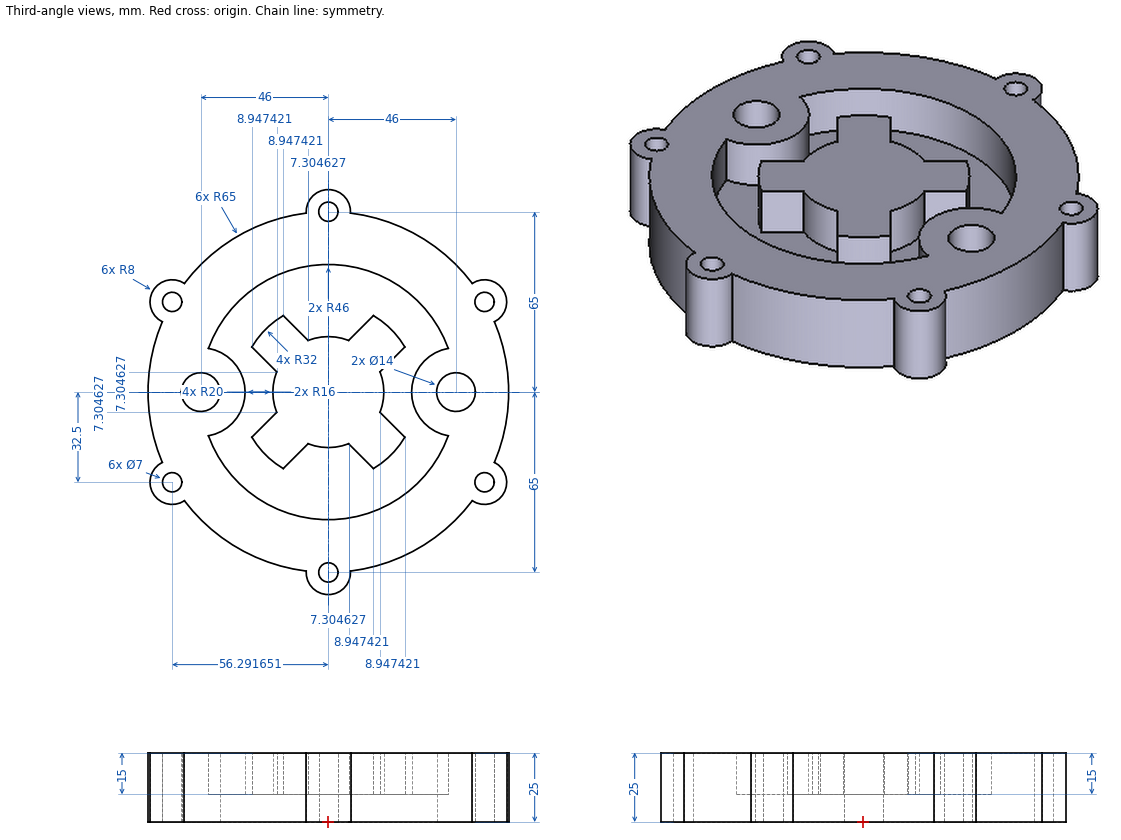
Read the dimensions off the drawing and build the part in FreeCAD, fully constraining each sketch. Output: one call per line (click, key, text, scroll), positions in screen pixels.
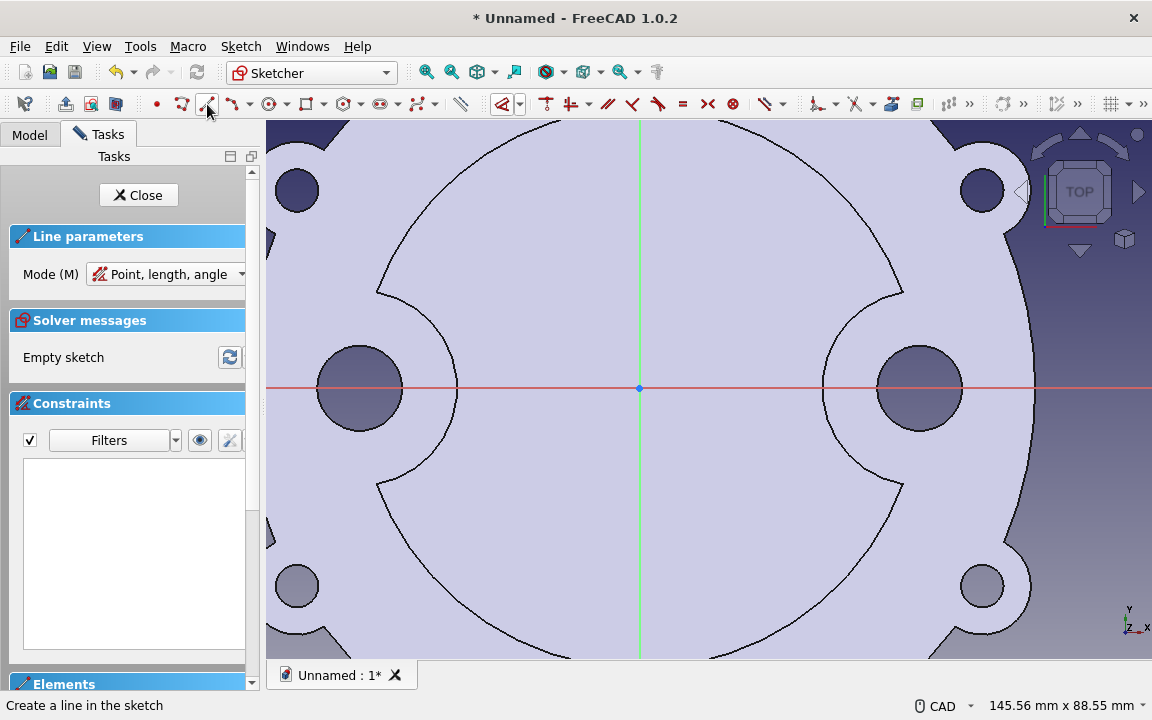
click(595, 275)
click(541, 220)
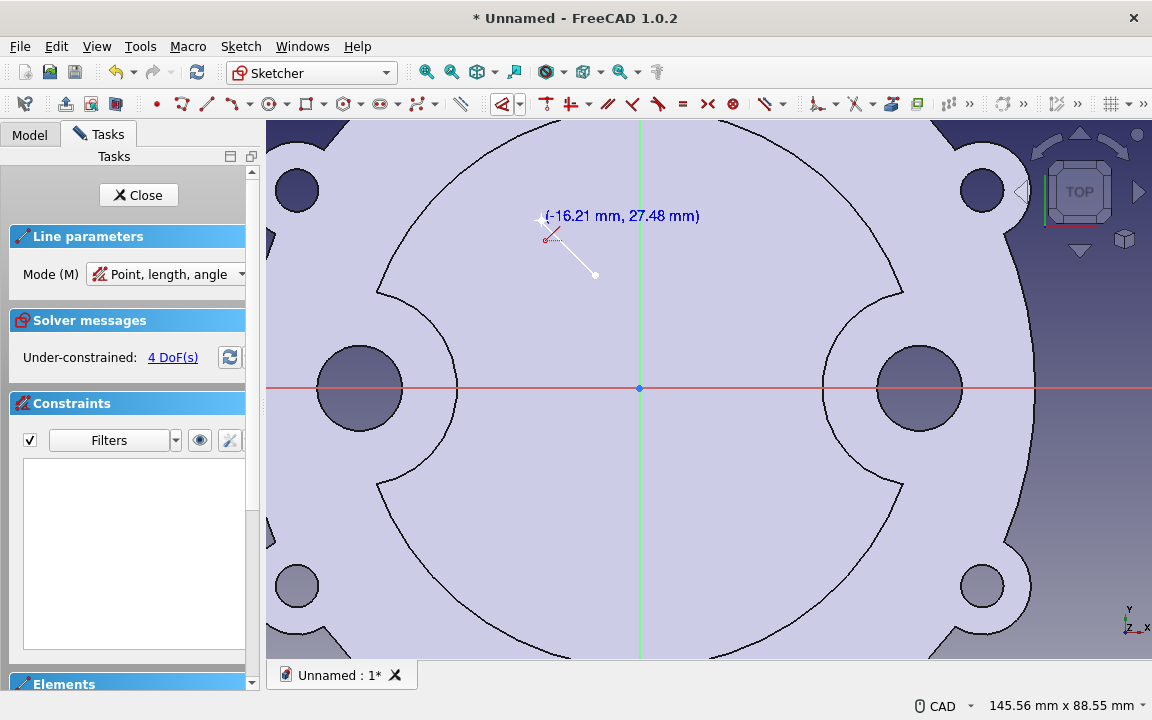
click(472, 289)
click(526, 344)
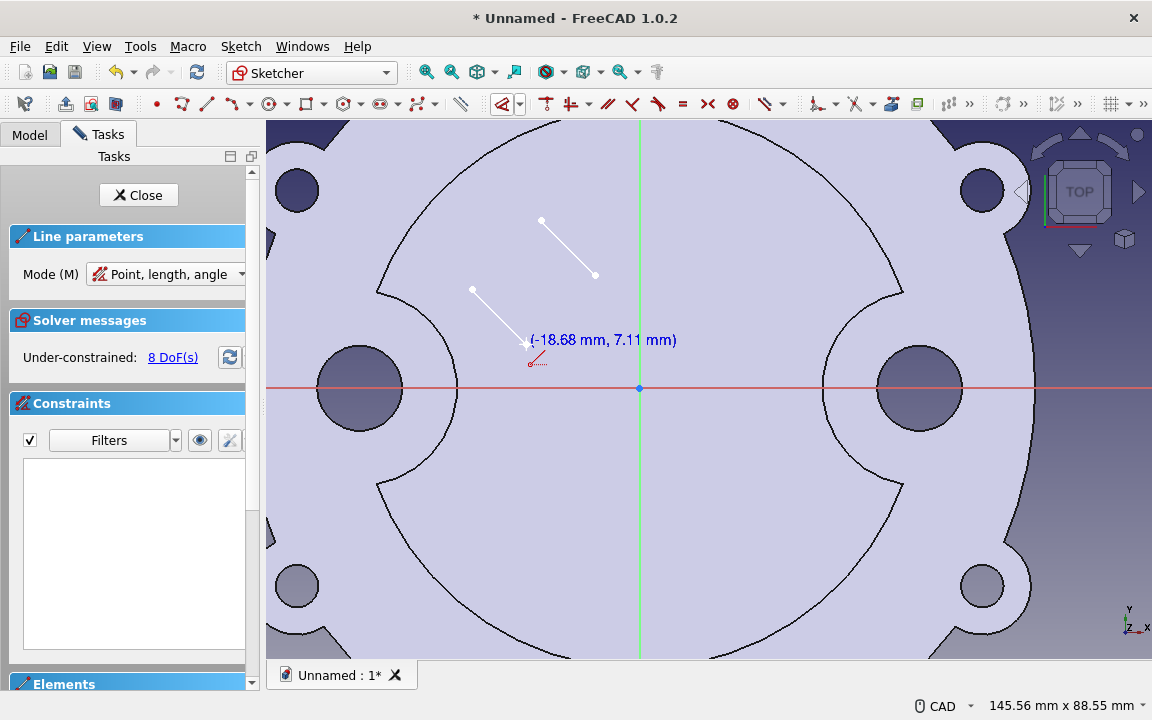
click(526, 433)
click(472, 487)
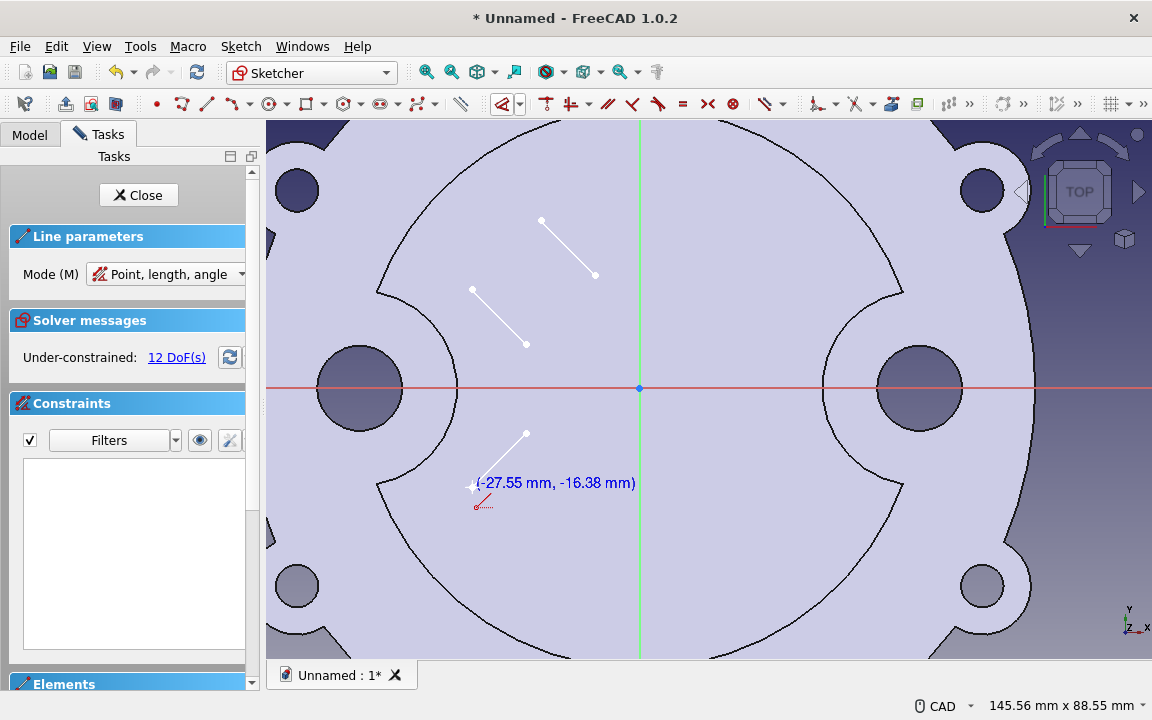
click(541, 556)
click(595, 502)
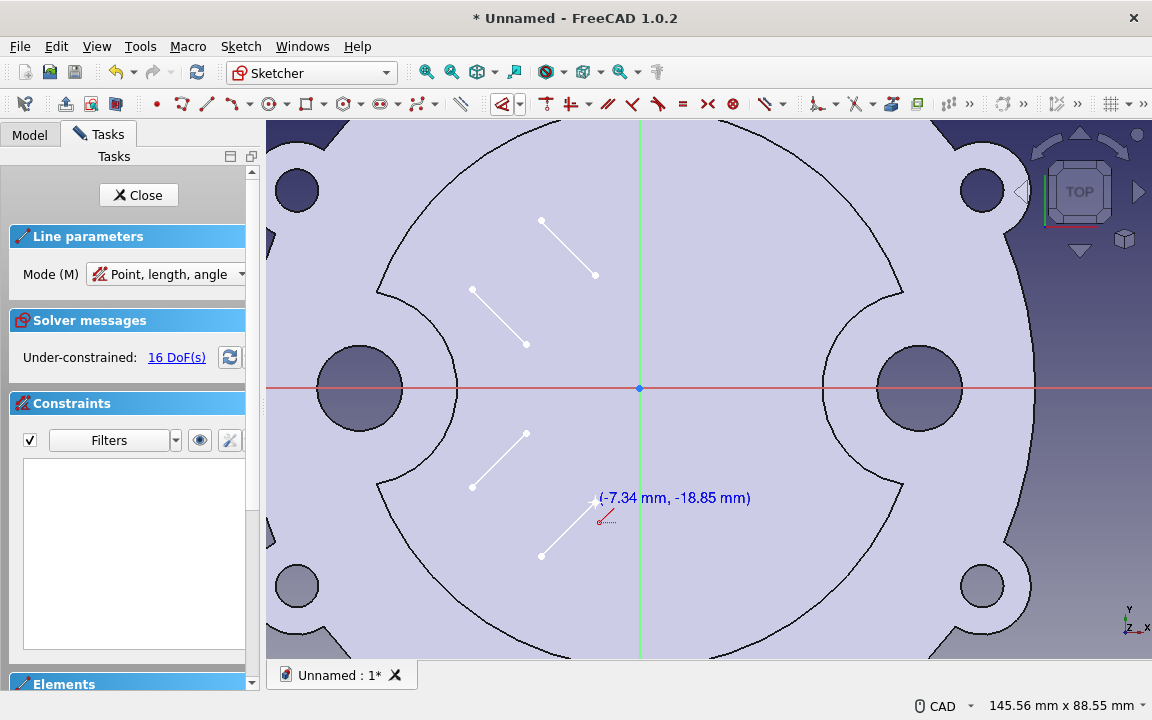
click(684, 502)
click(739, 556)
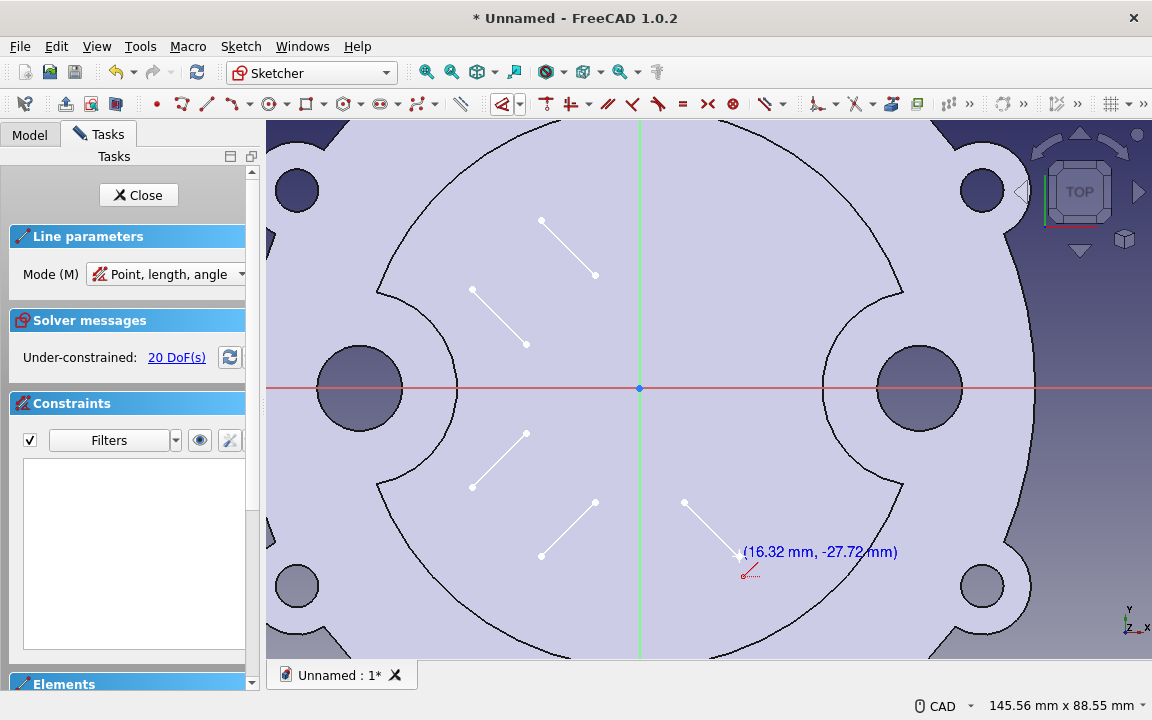
click(807, 487)
click(753, 433)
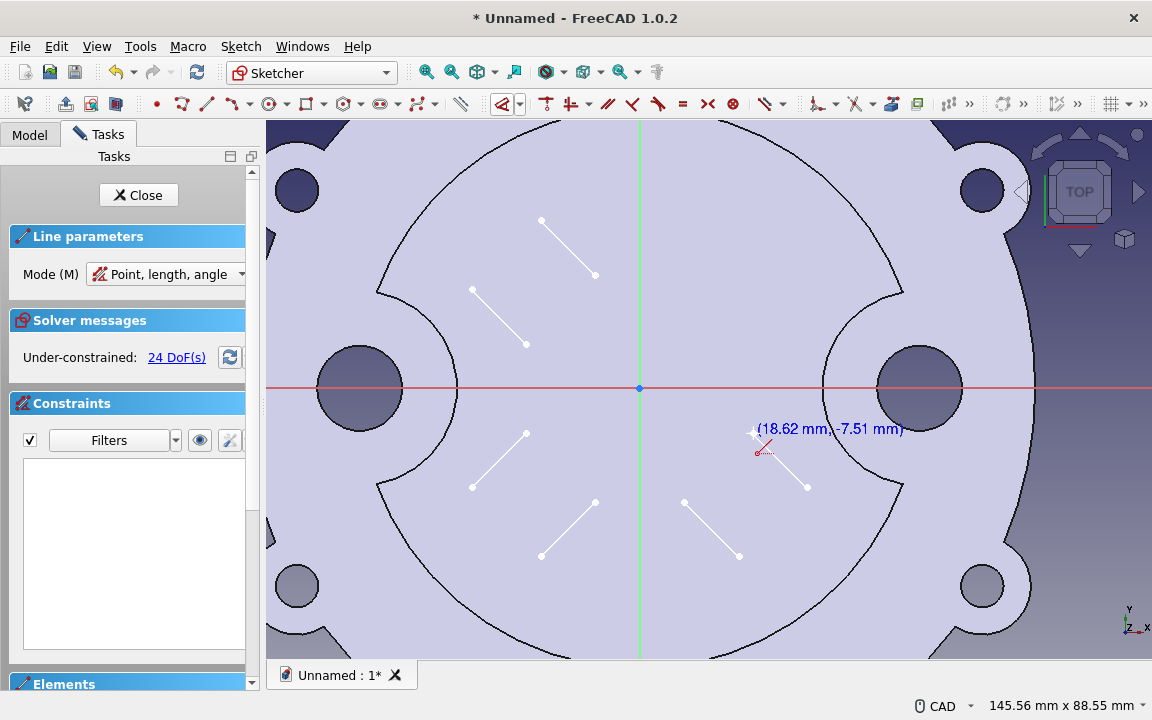
click(753, 344)
click(807, 289)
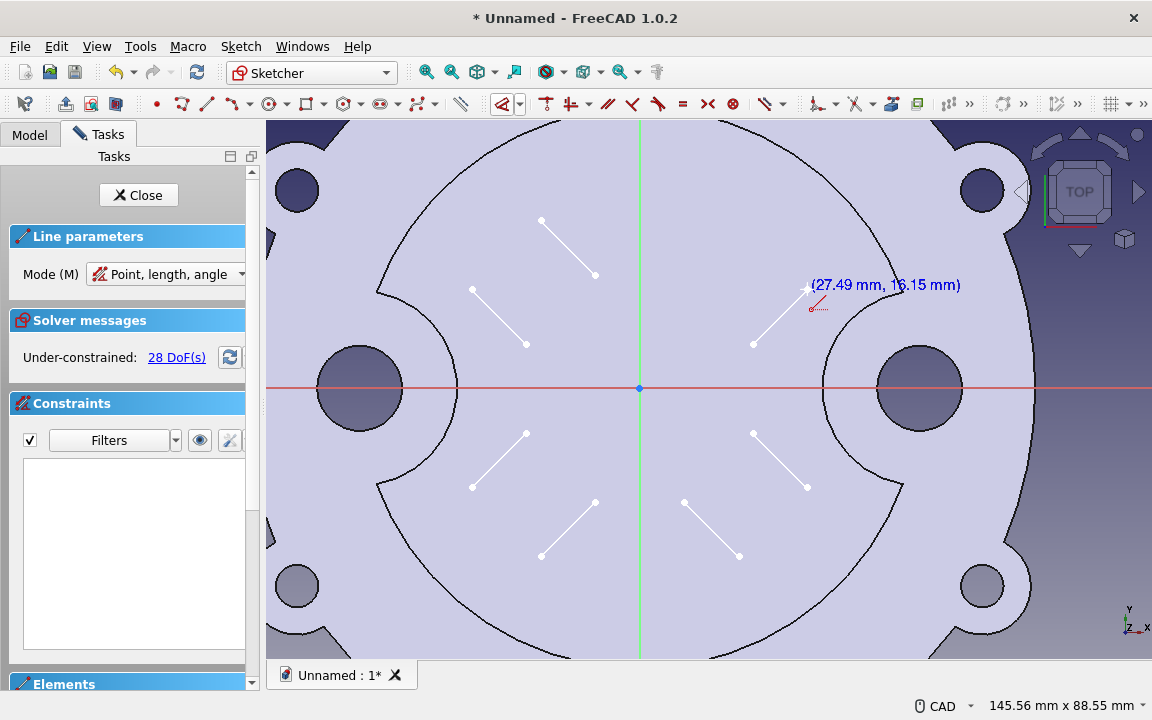
click(739, 220)
click(684, 275)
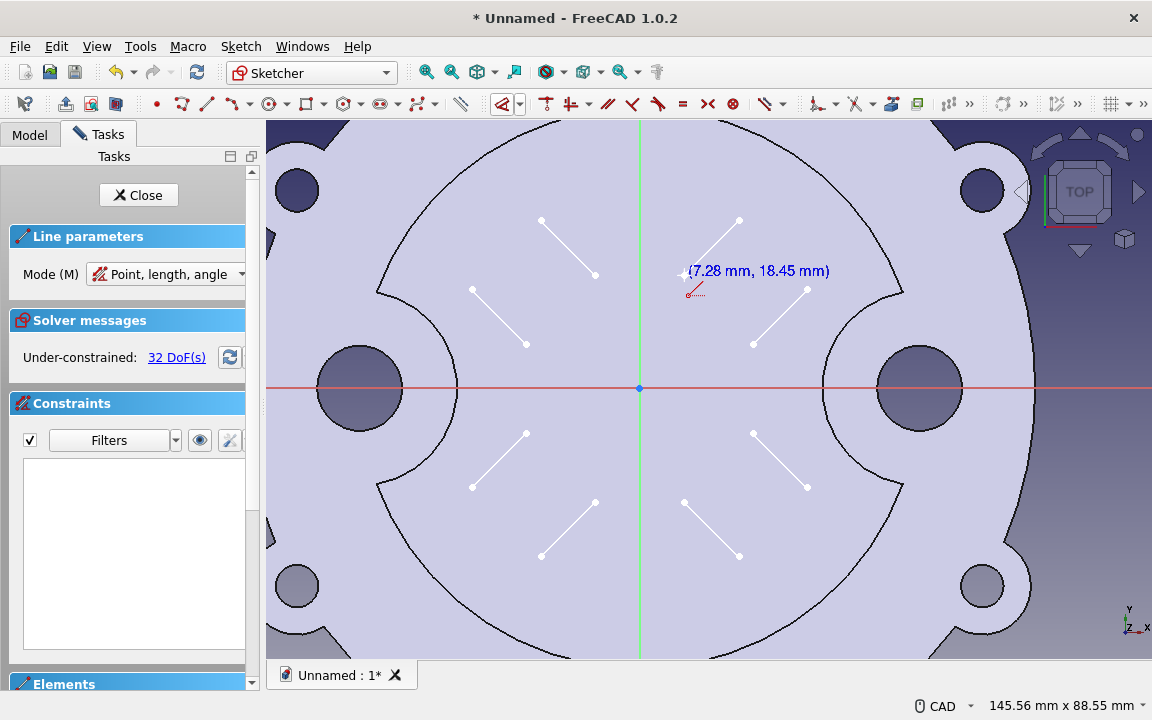
click(232, 104)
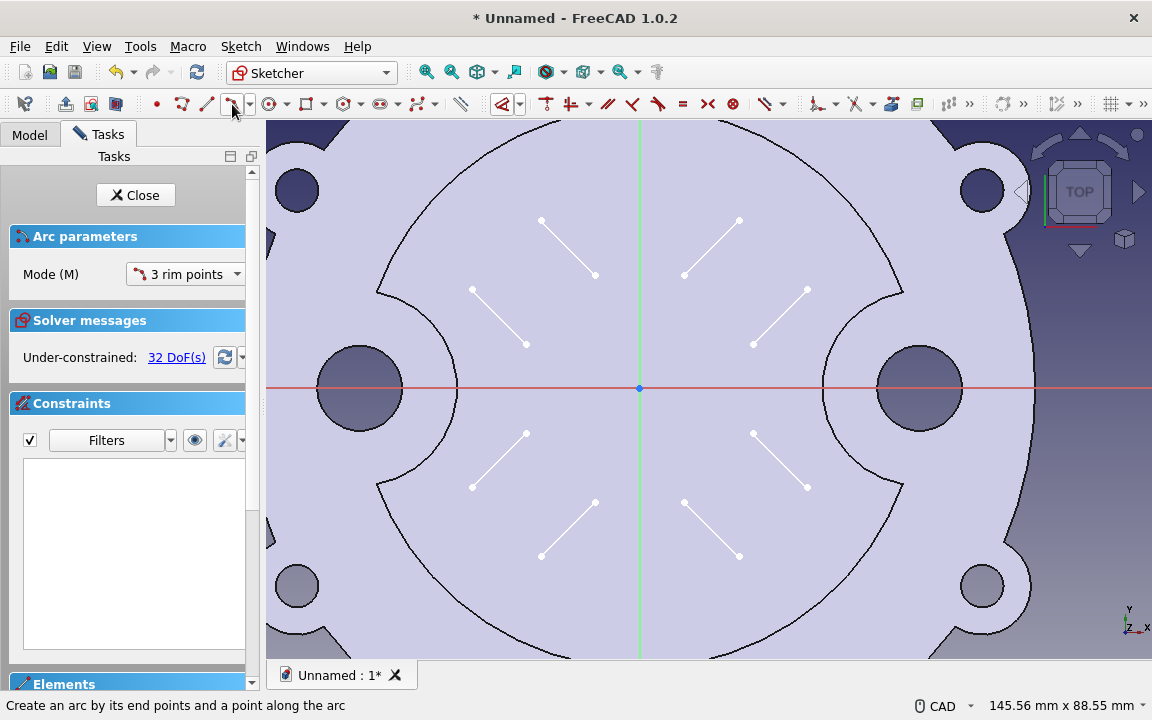
click(541, 221)
click(472, 290)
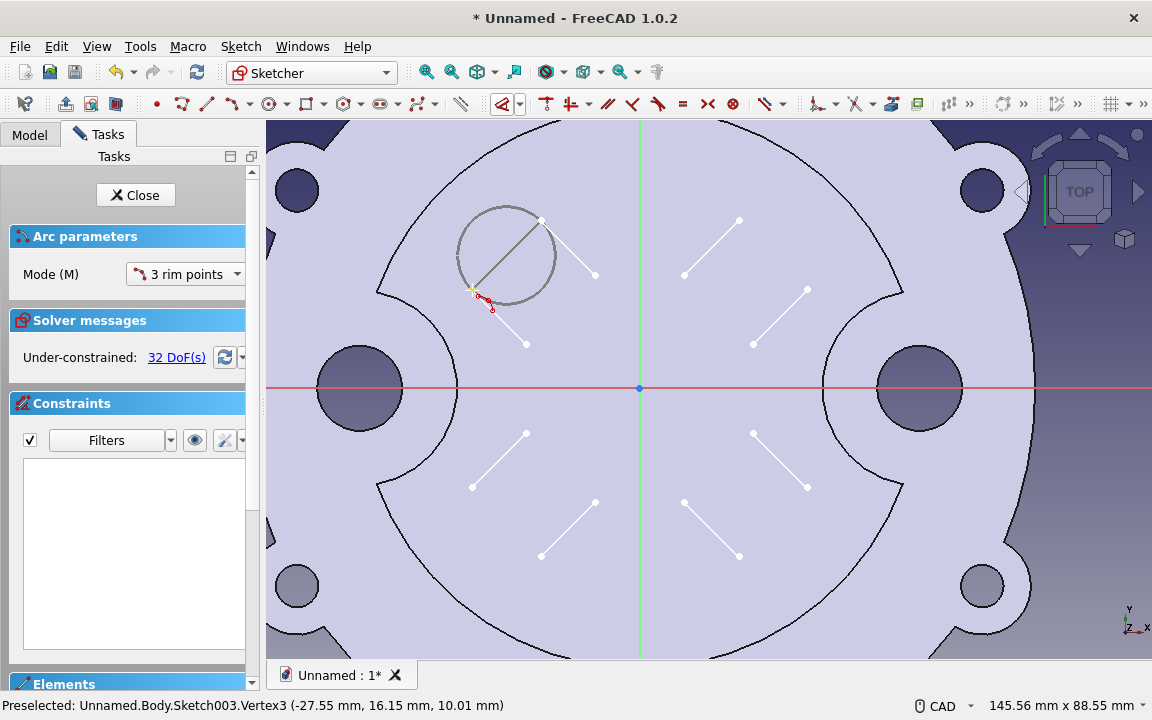
scroll(502, 251, up, 5)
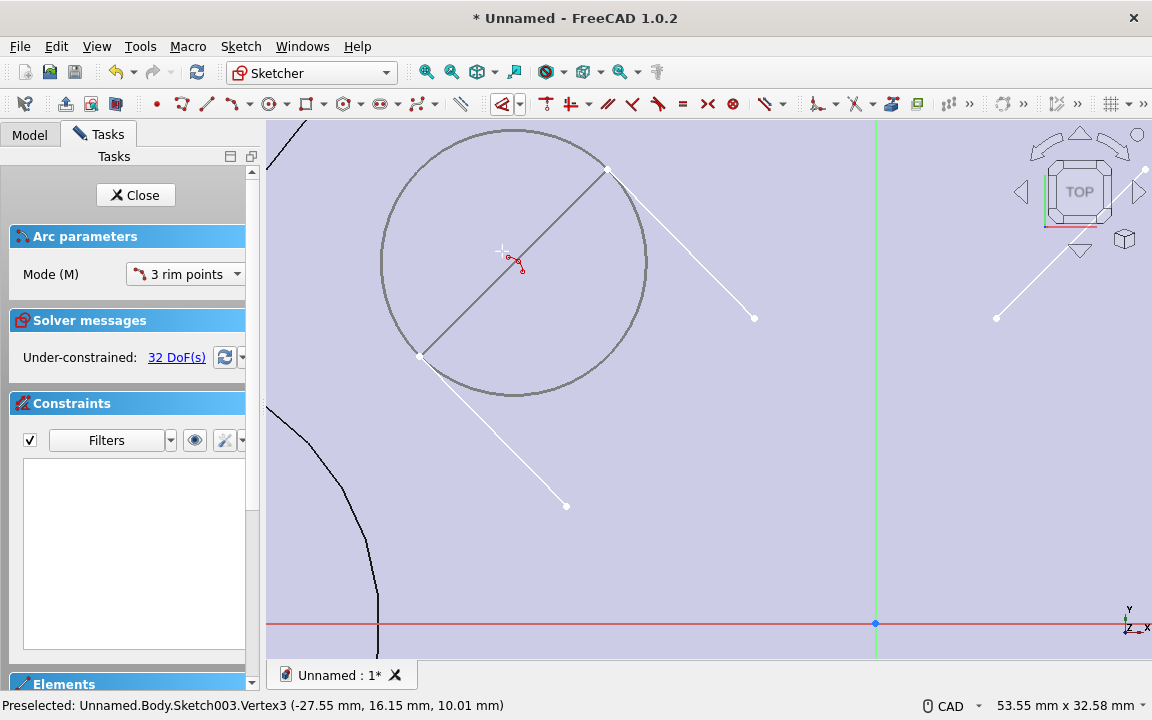
click(501, 249)